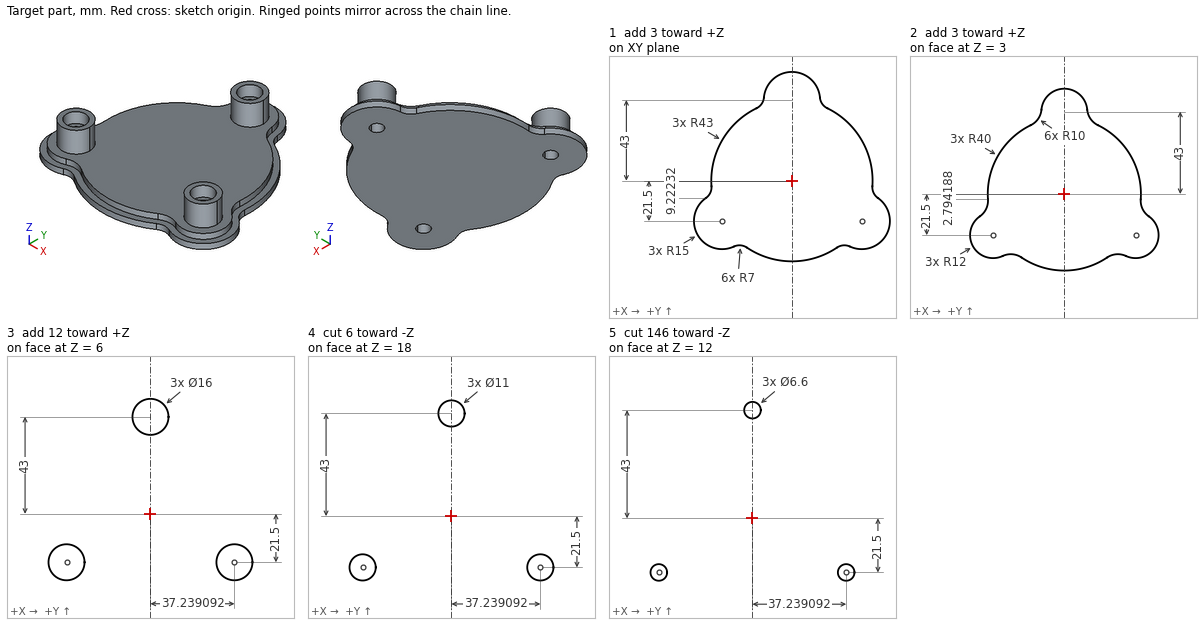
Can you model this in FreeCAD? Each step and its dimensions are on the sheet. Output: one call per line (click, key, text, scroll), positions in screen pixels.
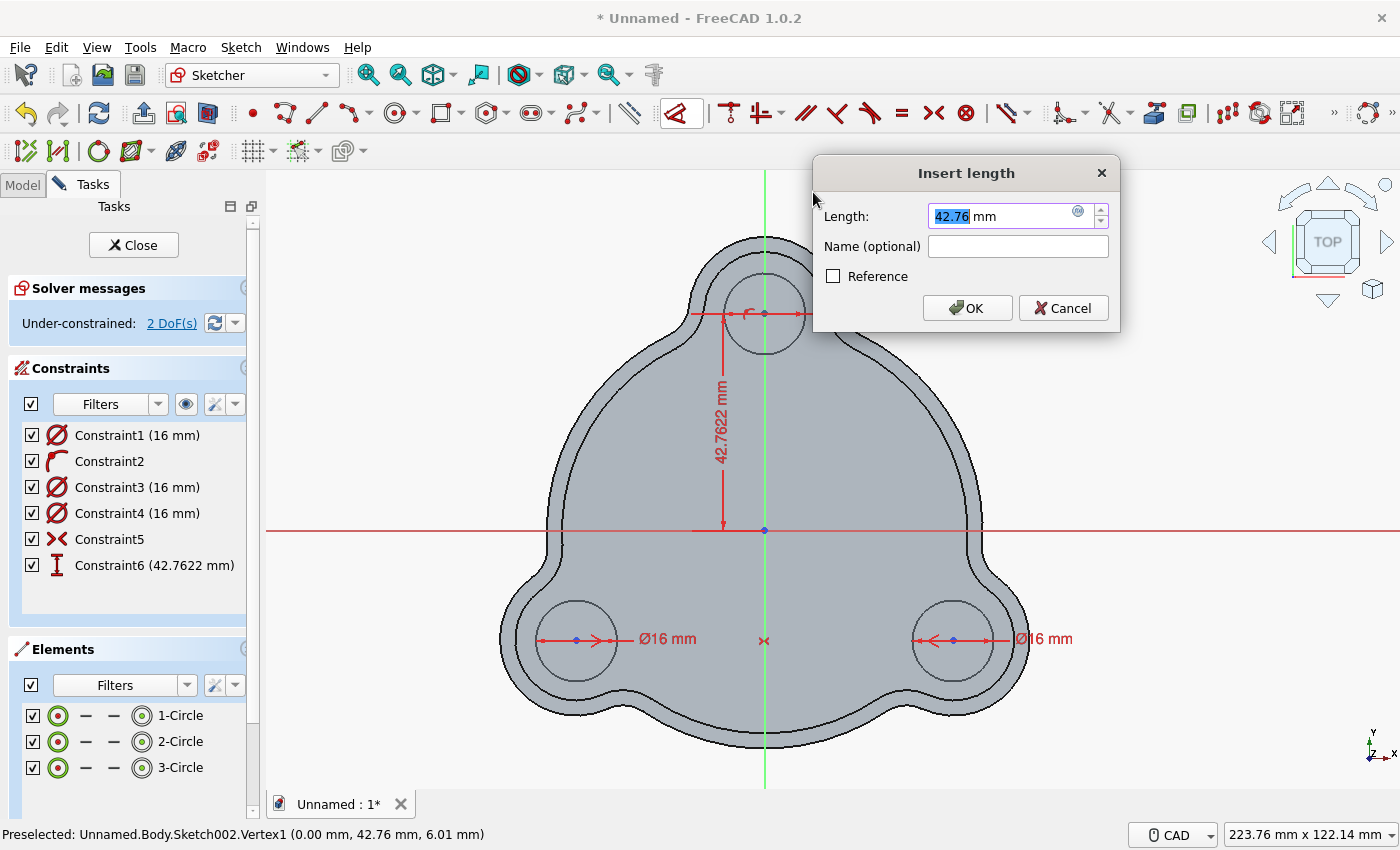
text(43)
key(Return)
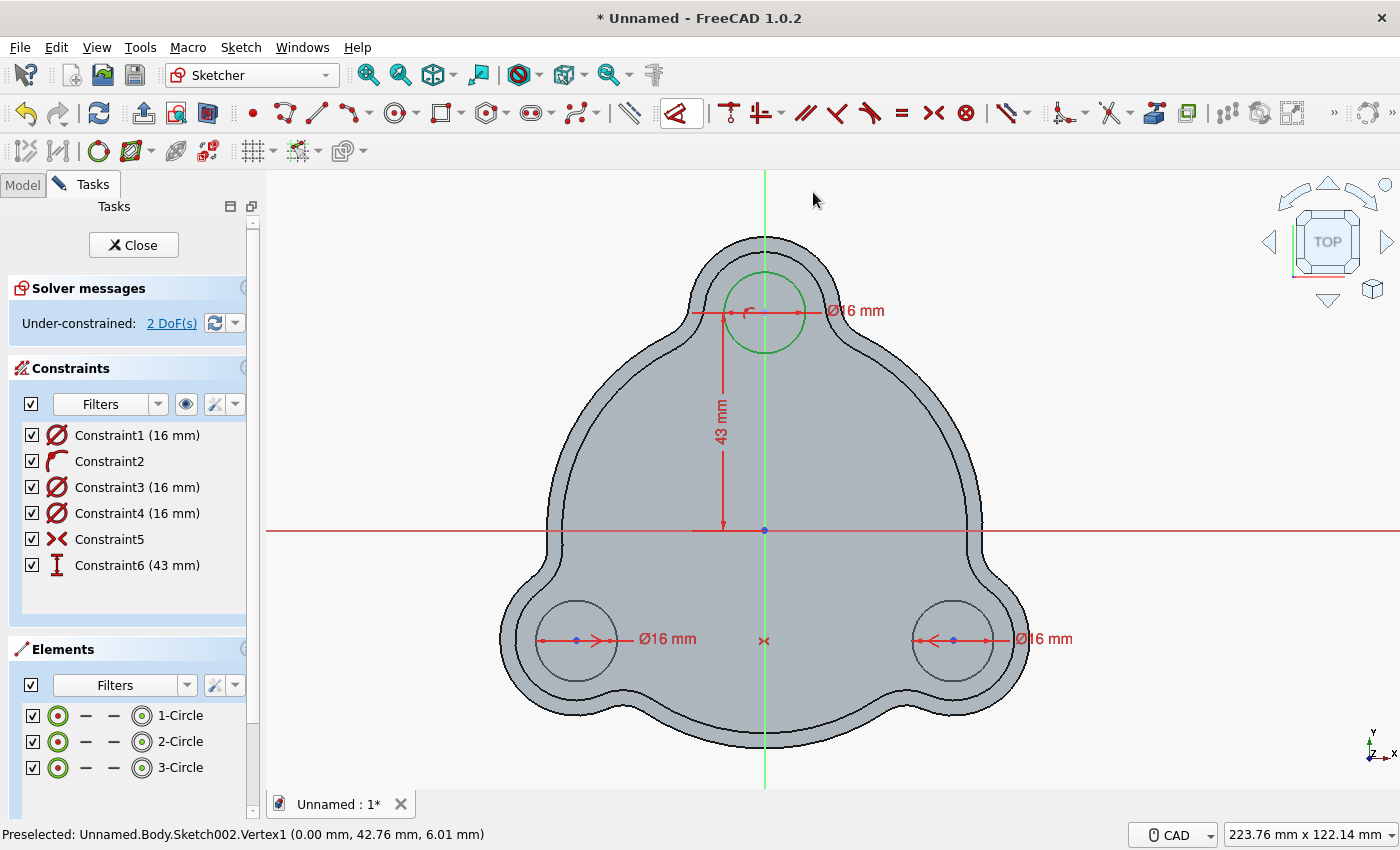
click(953, 641)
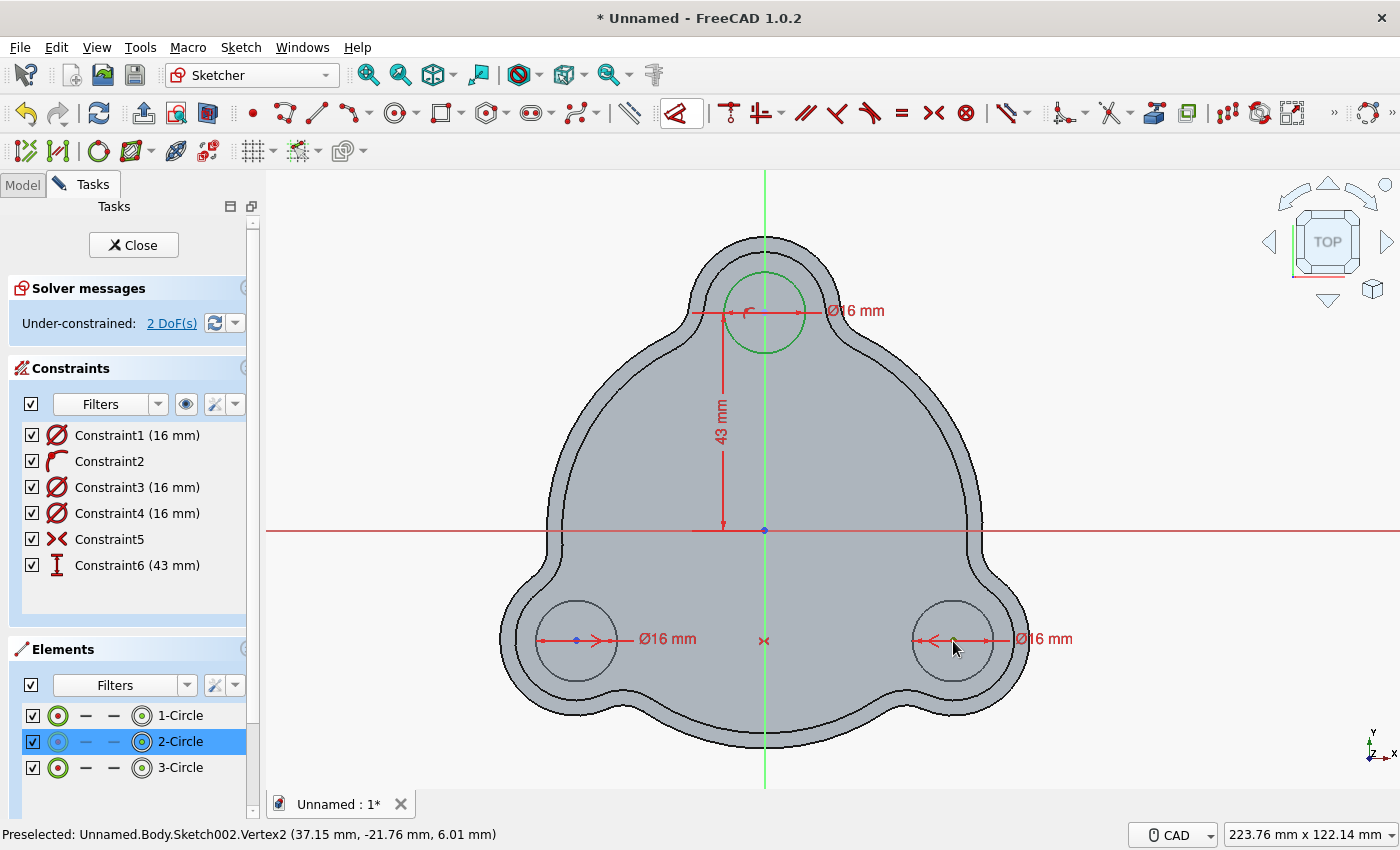
click(698, 114)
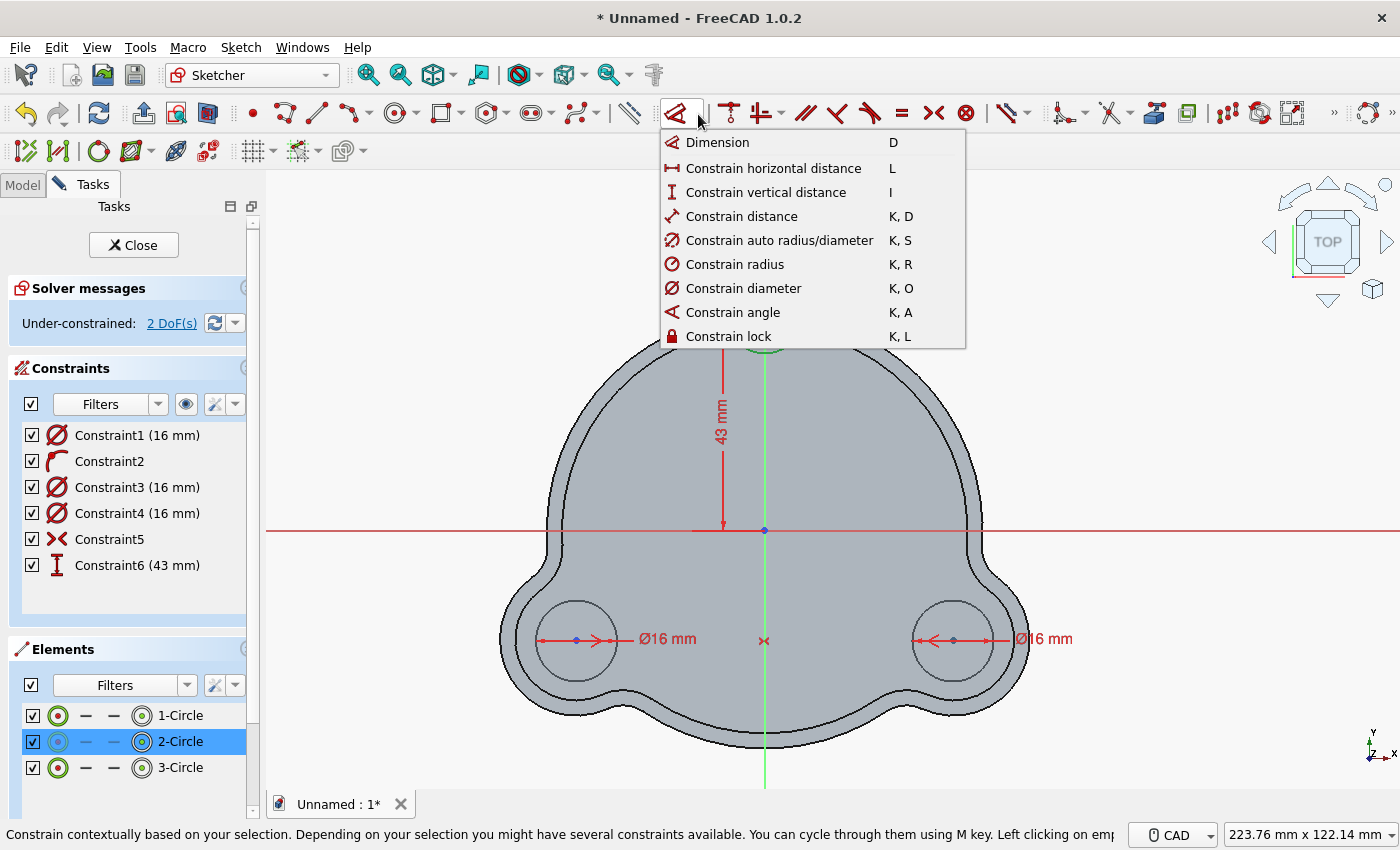
click(813, 192)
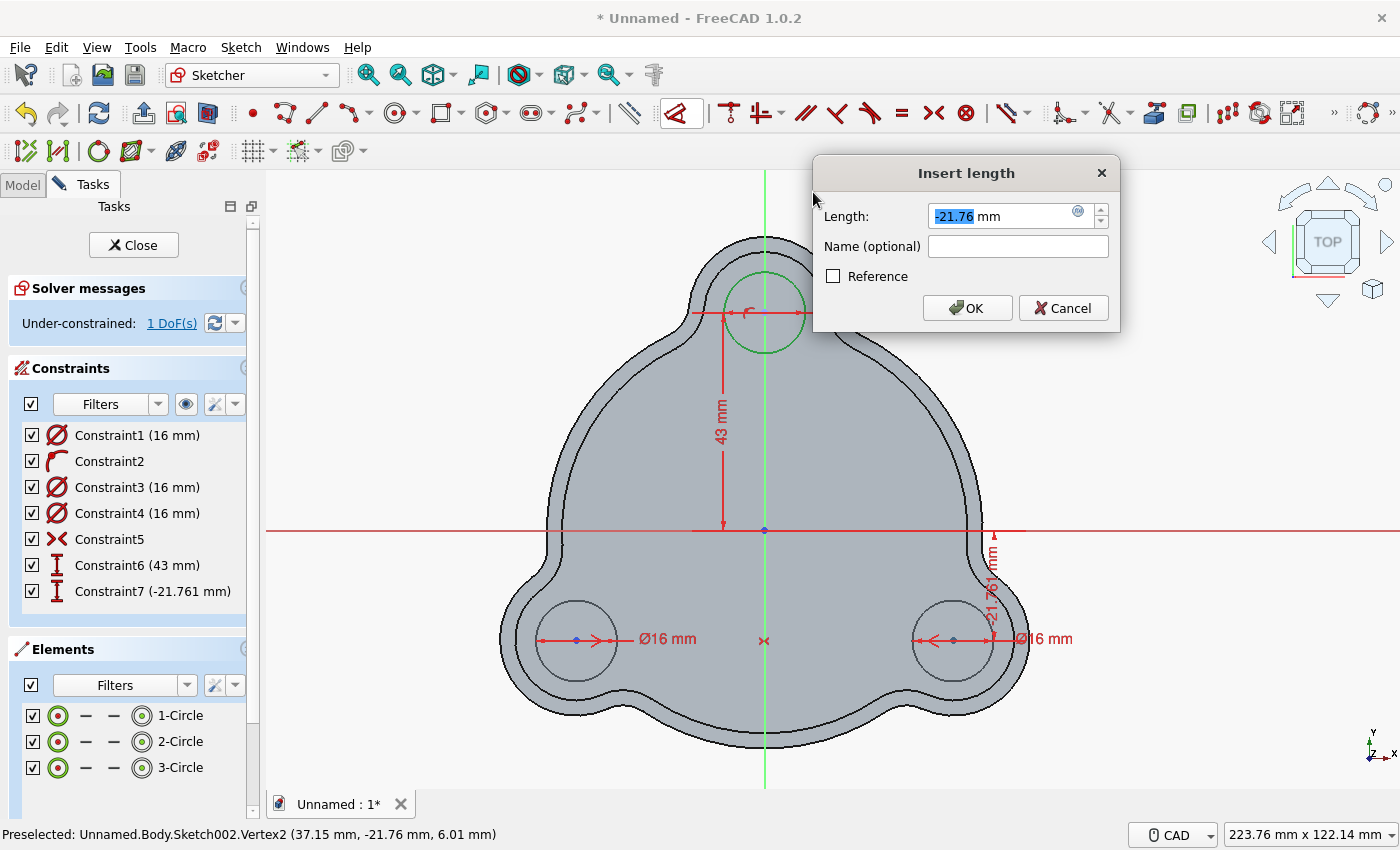
text(-21.5)
key(Return)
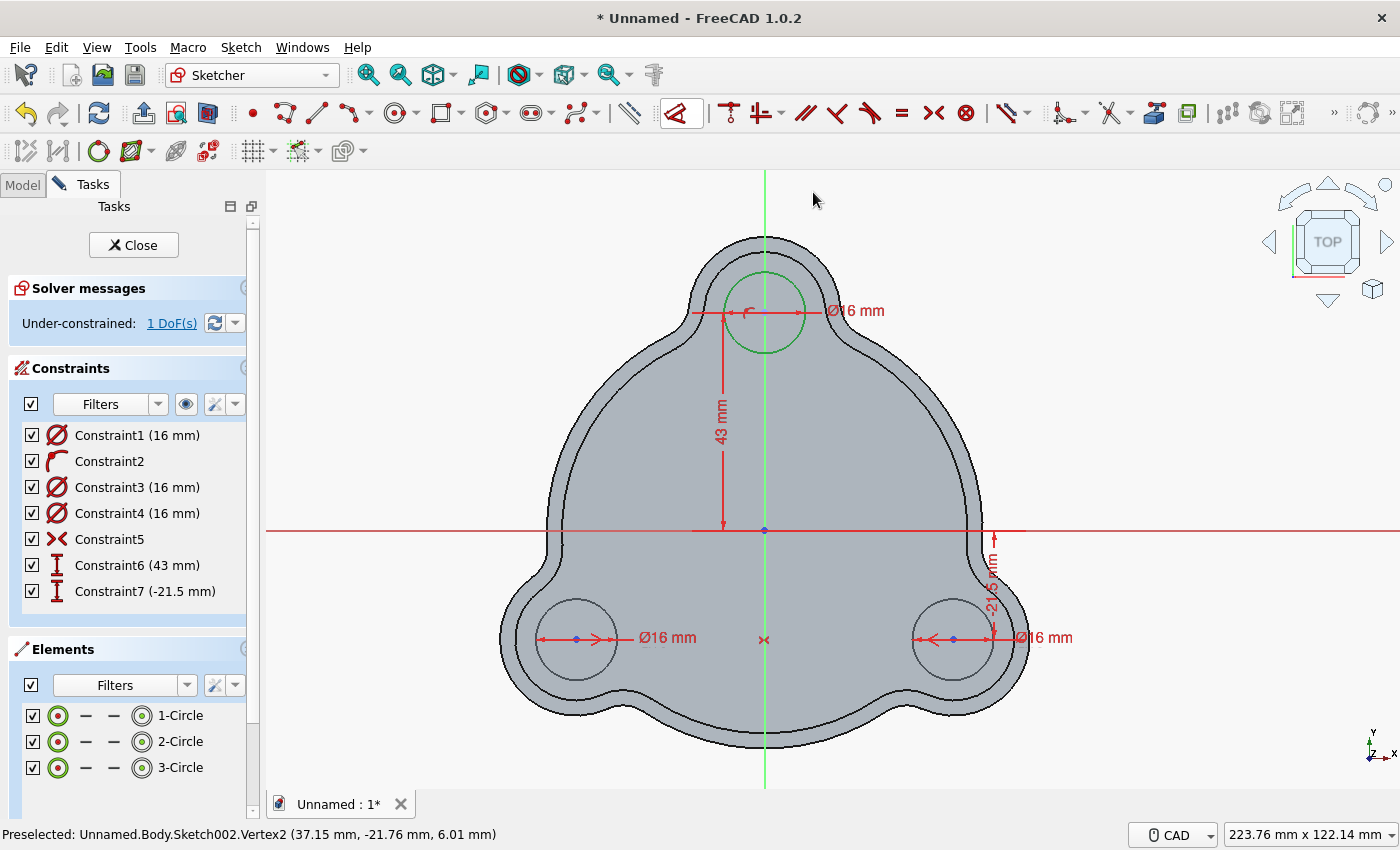
click(953, 640)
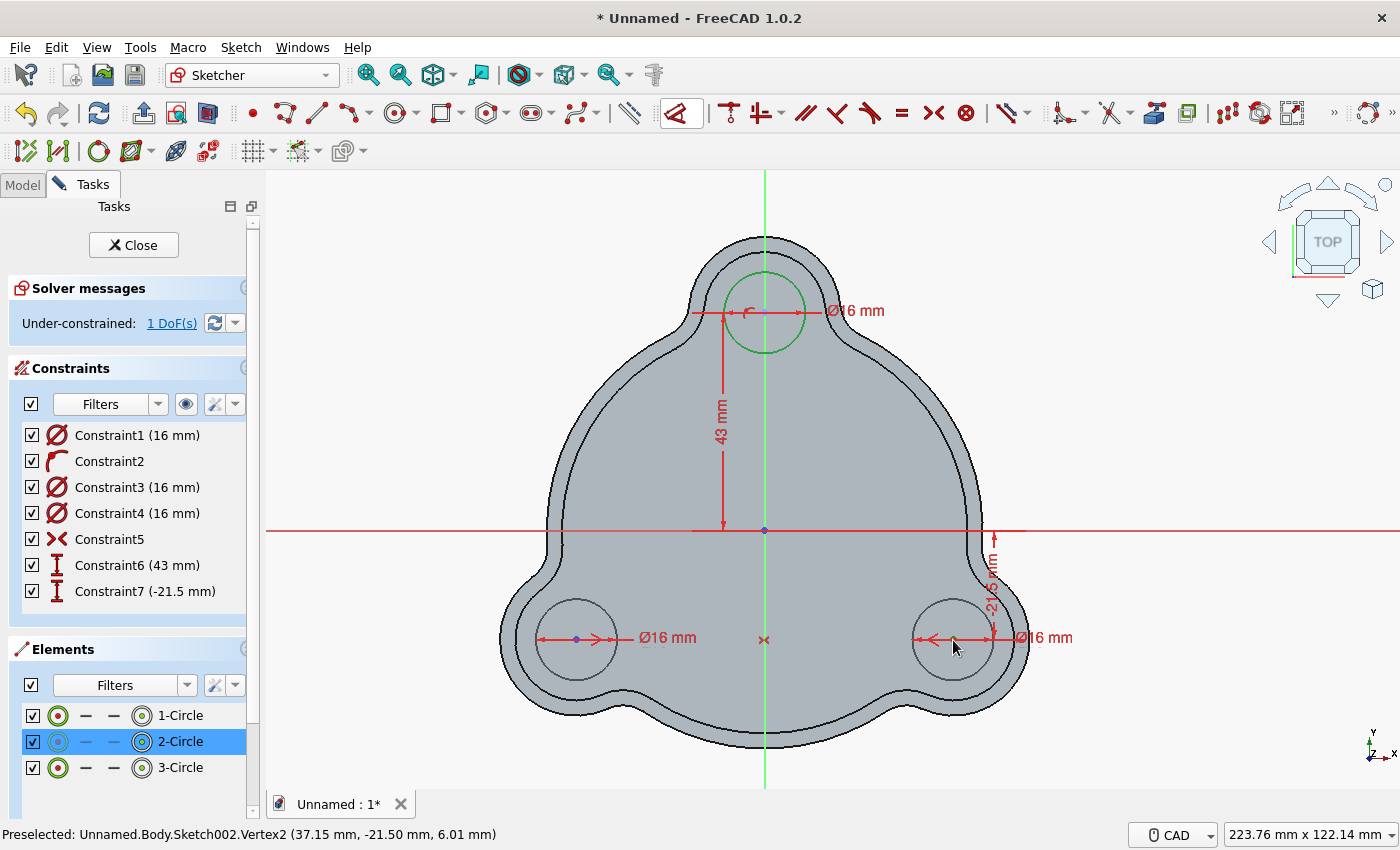
click(698, 114)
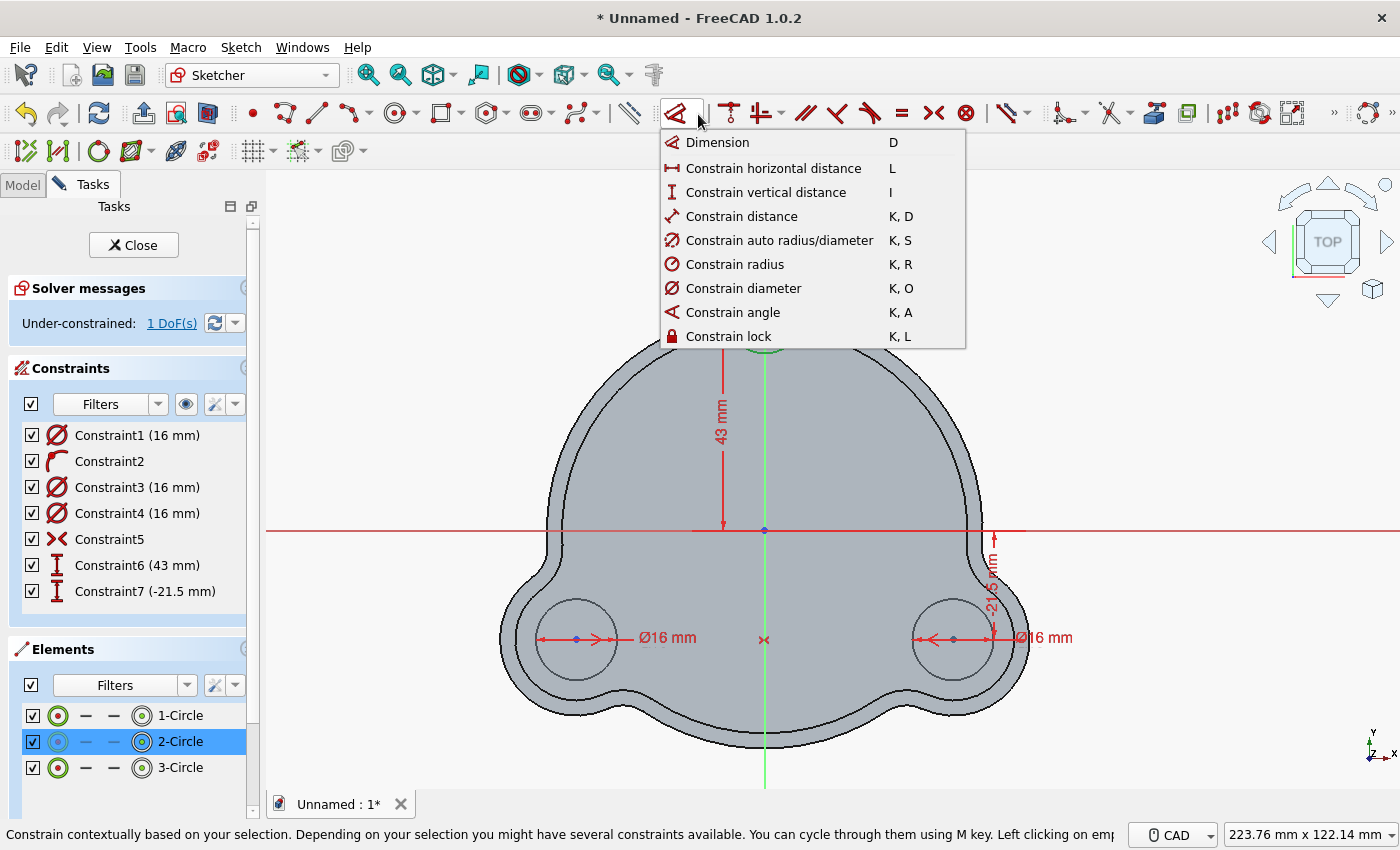
click(813, 168)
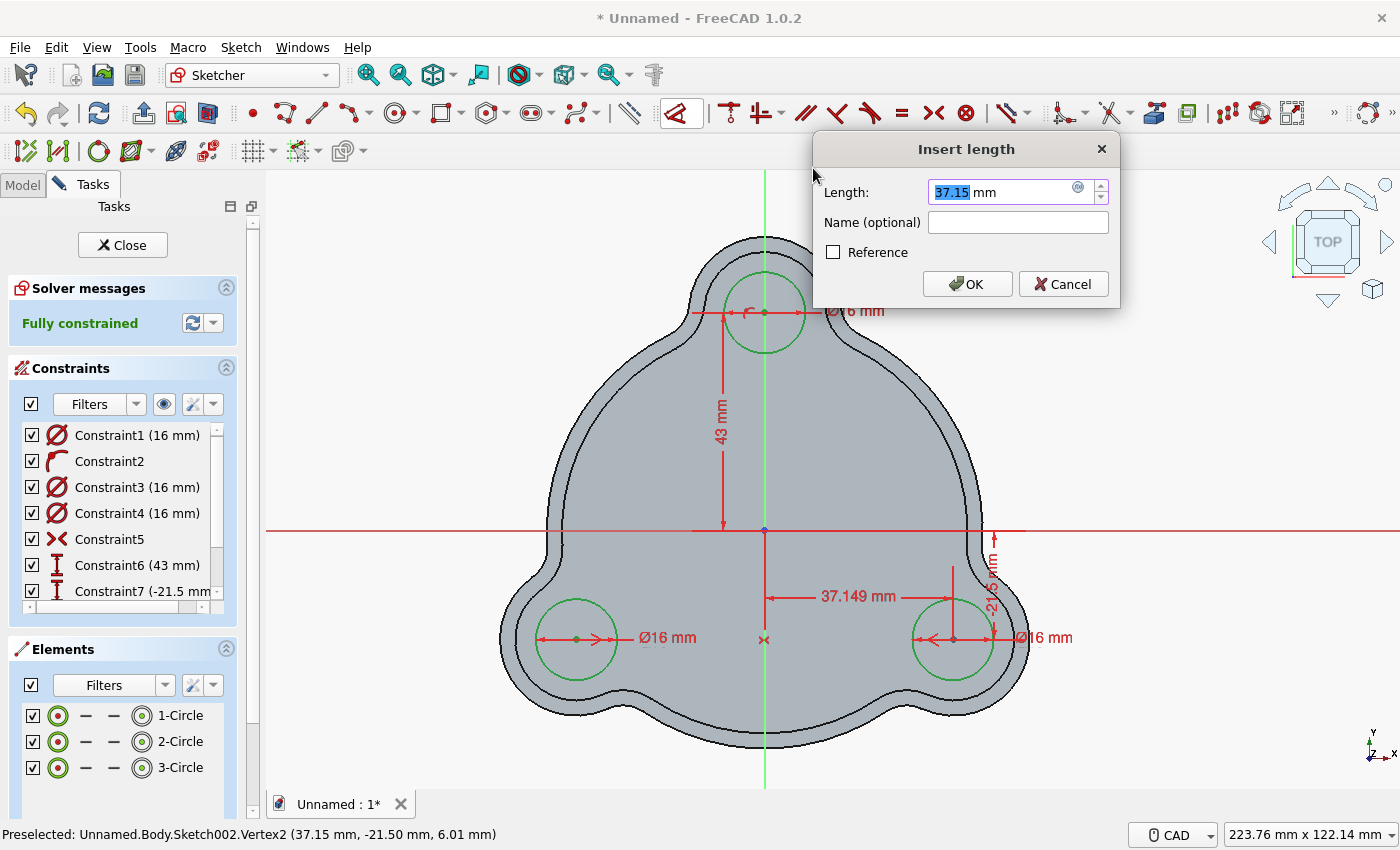
text(37.239092)
key(Return)